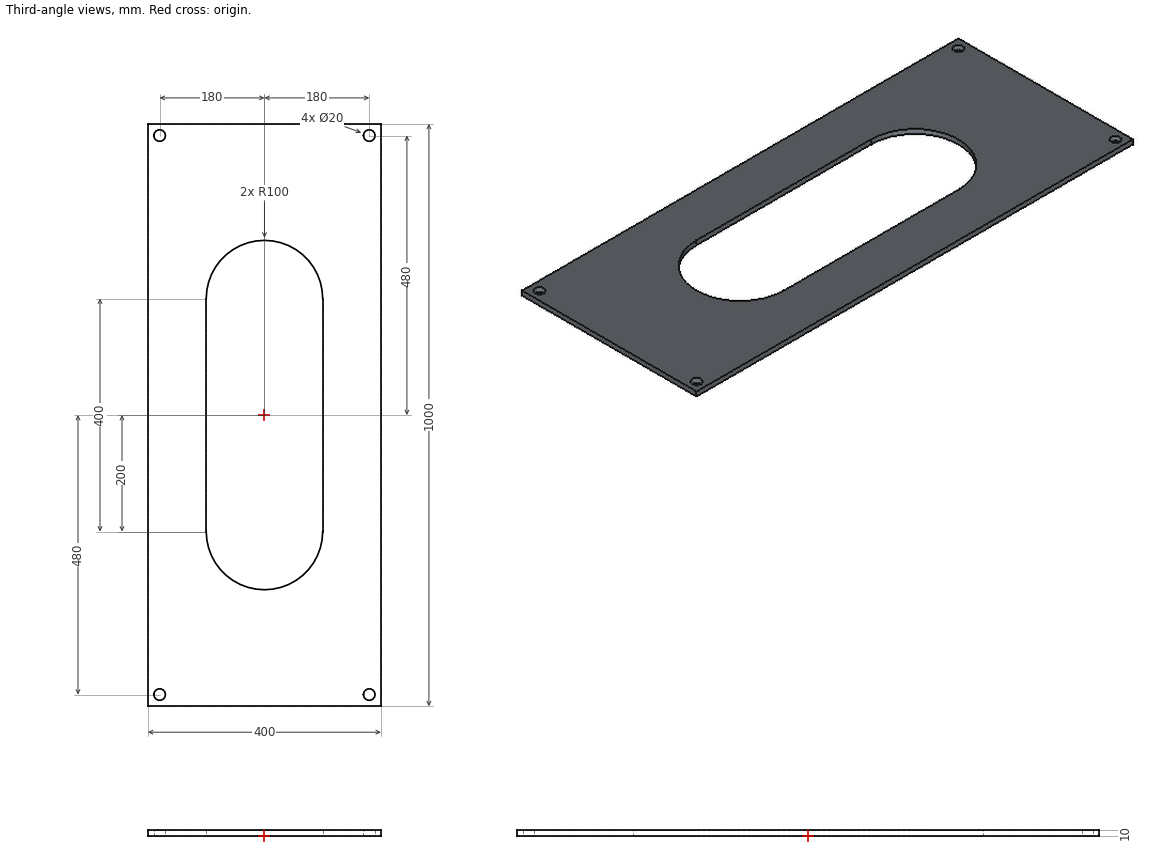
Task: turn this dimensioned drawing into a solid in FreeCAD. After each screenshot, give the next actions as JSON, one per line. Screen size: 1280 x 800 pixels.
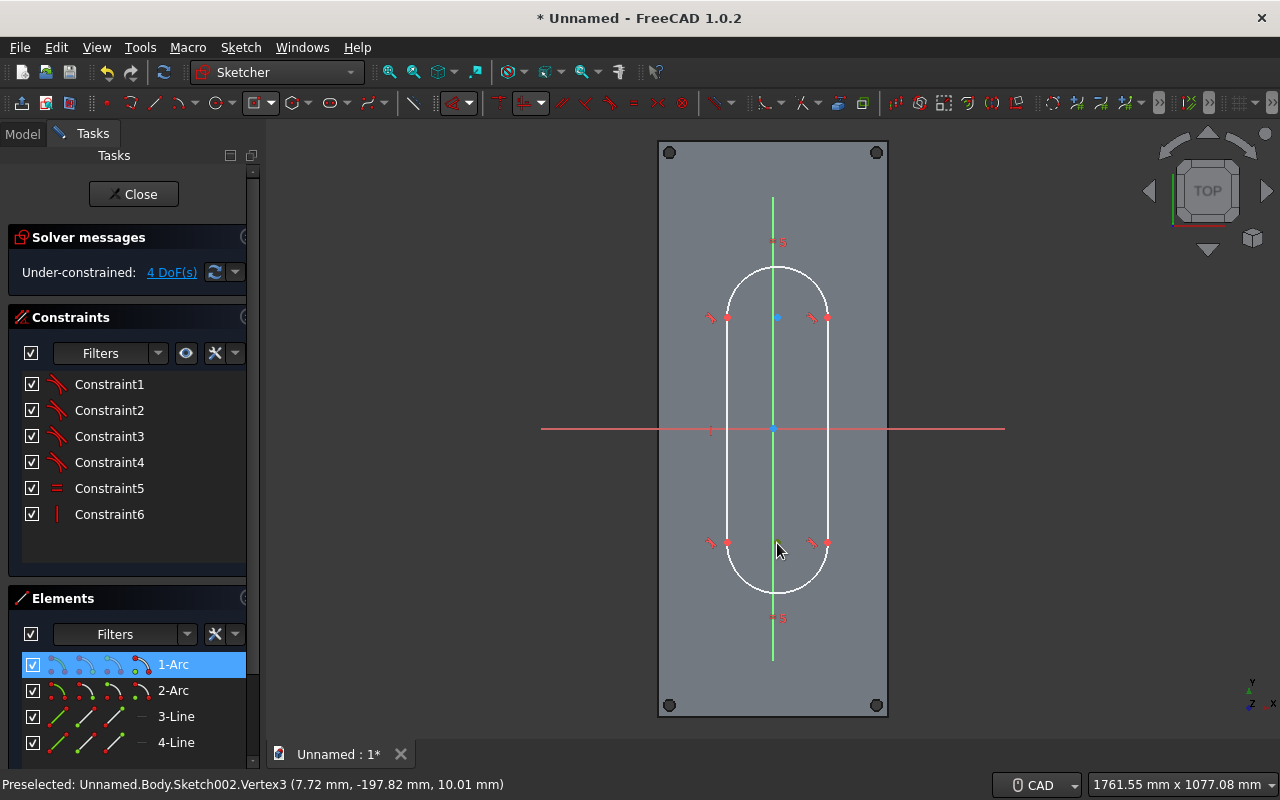
{"action": "left_click", "coordinate": [773, 630]}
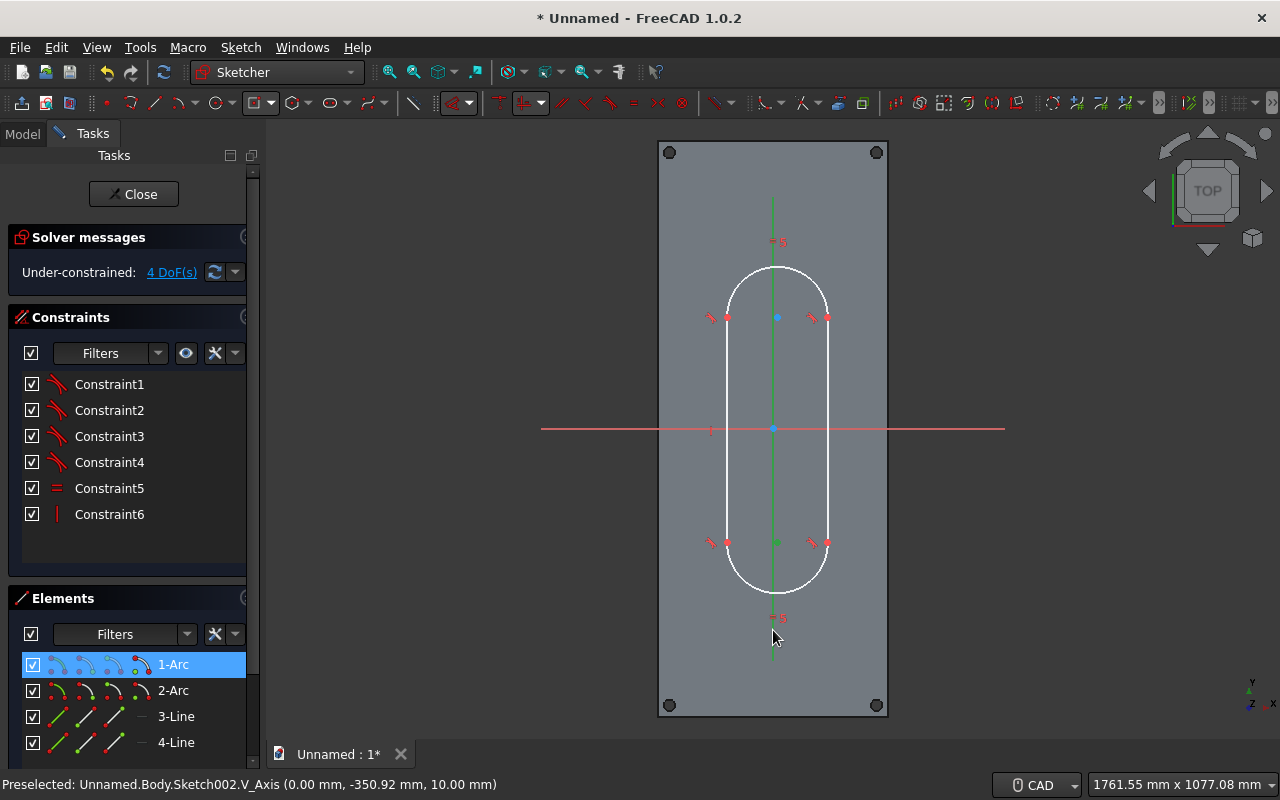
{"action": "left_click", "coordinate": [500, 104]}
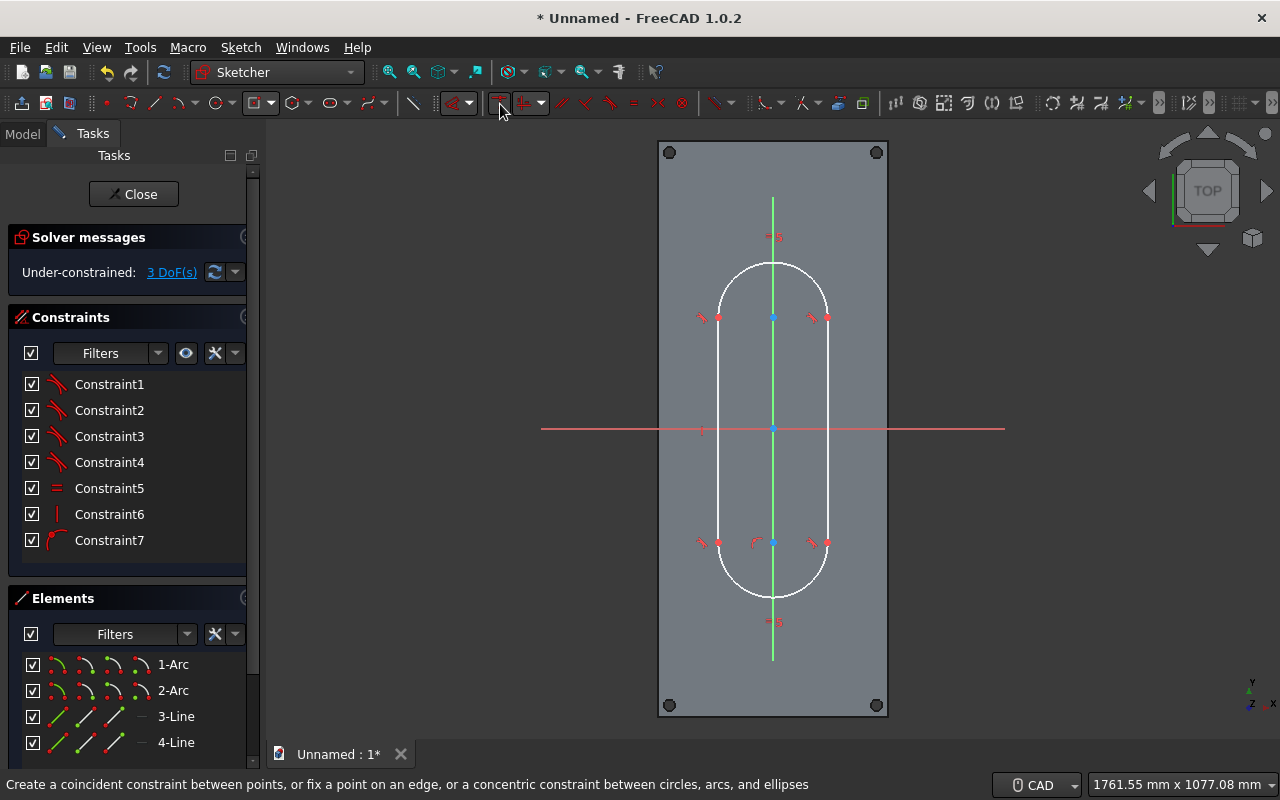
{"action": "left_click", "coordinate": [741, 587]}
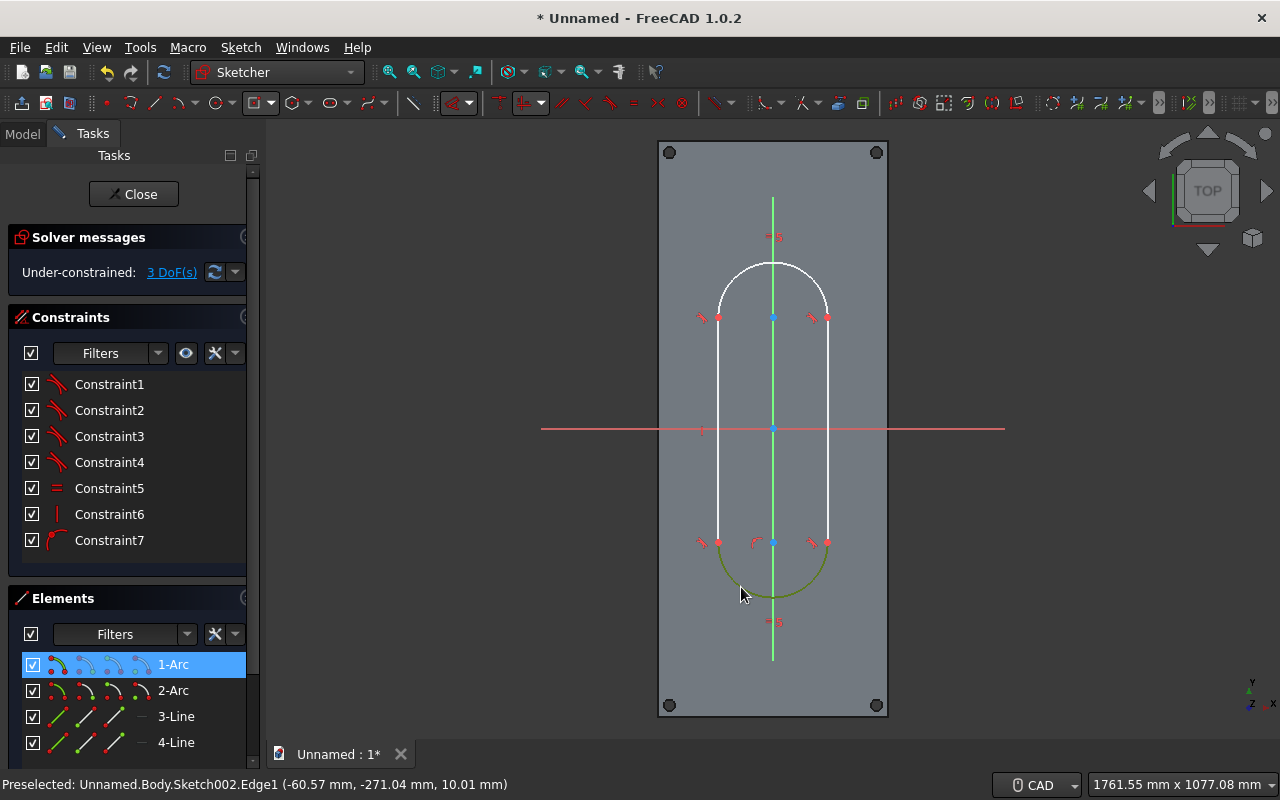
{"action": "left_click", "coordinate": [472, 104]}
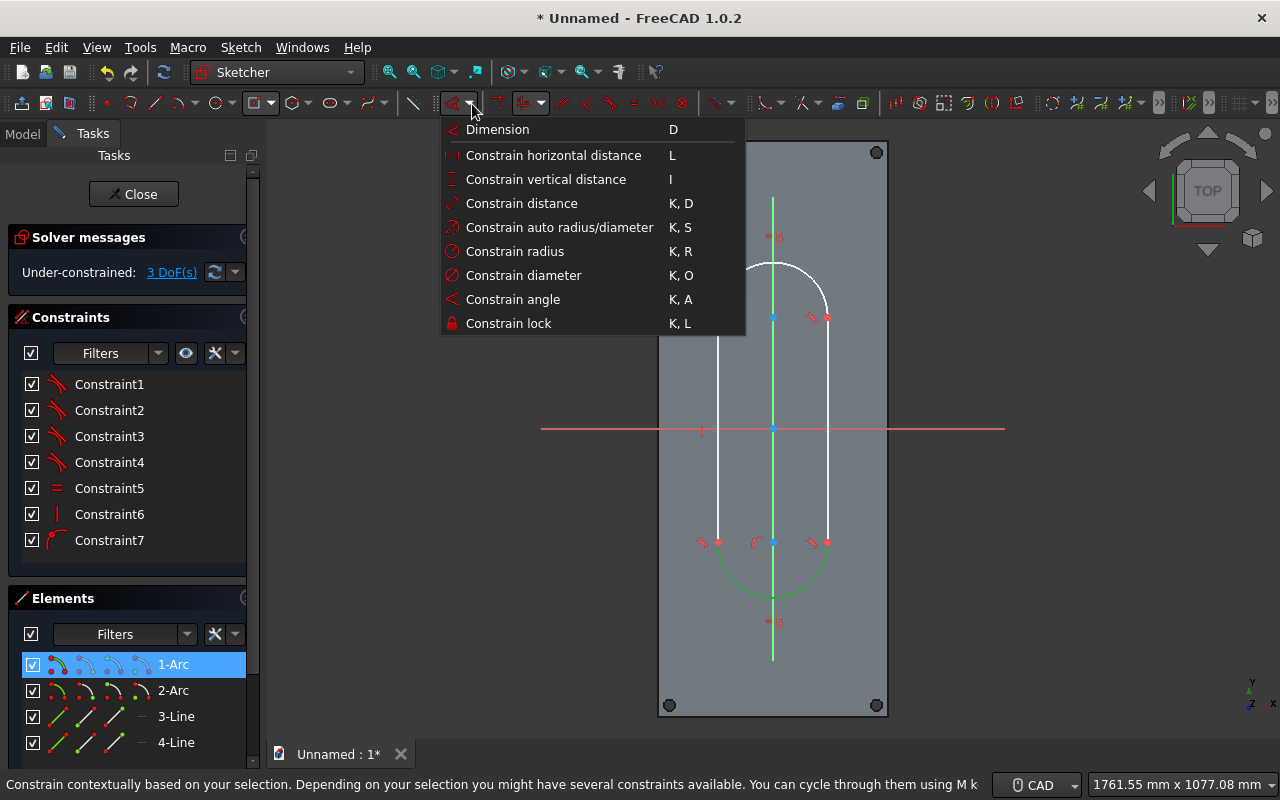
{"action": "left_click", "coordinate": [593, 251]}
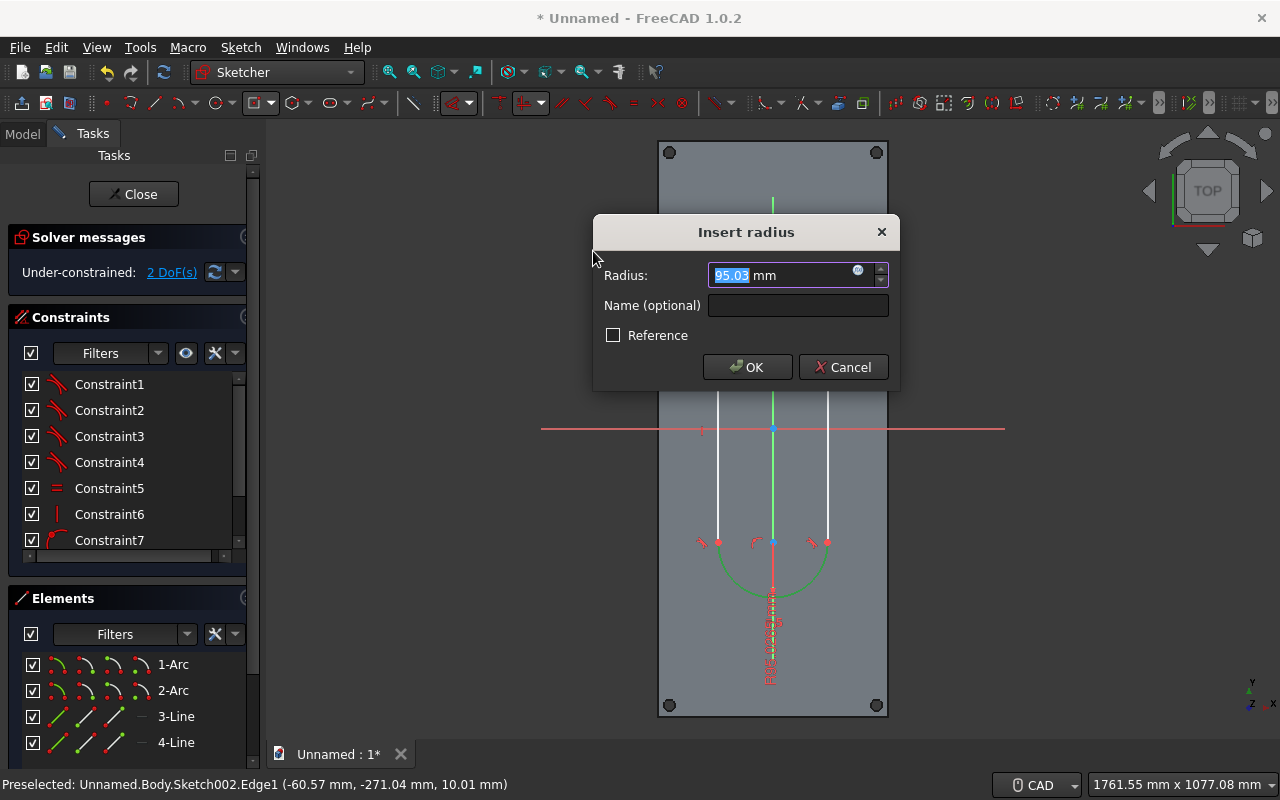
{"action": "type", "text": "100"}
{"action": "key", "text": "Return"}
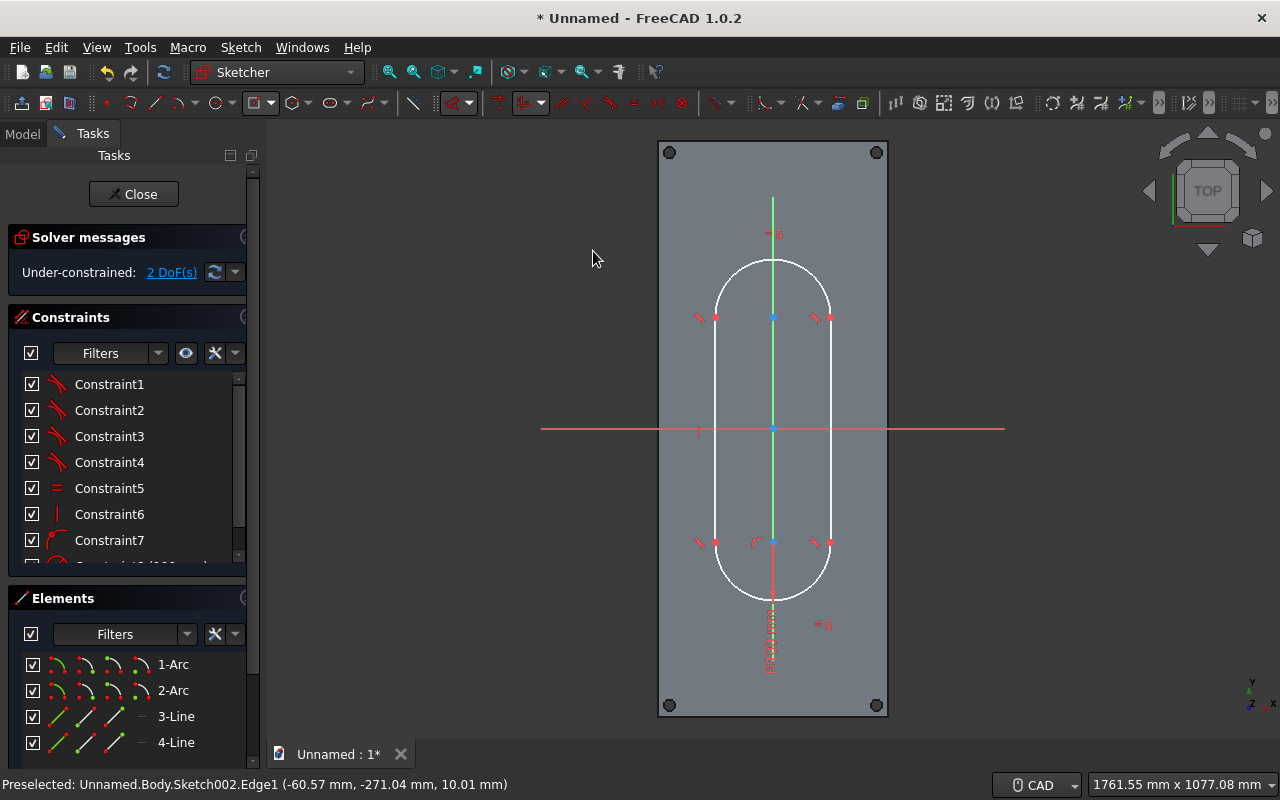
{"action": "left_click", "coordinate": [715, 475]}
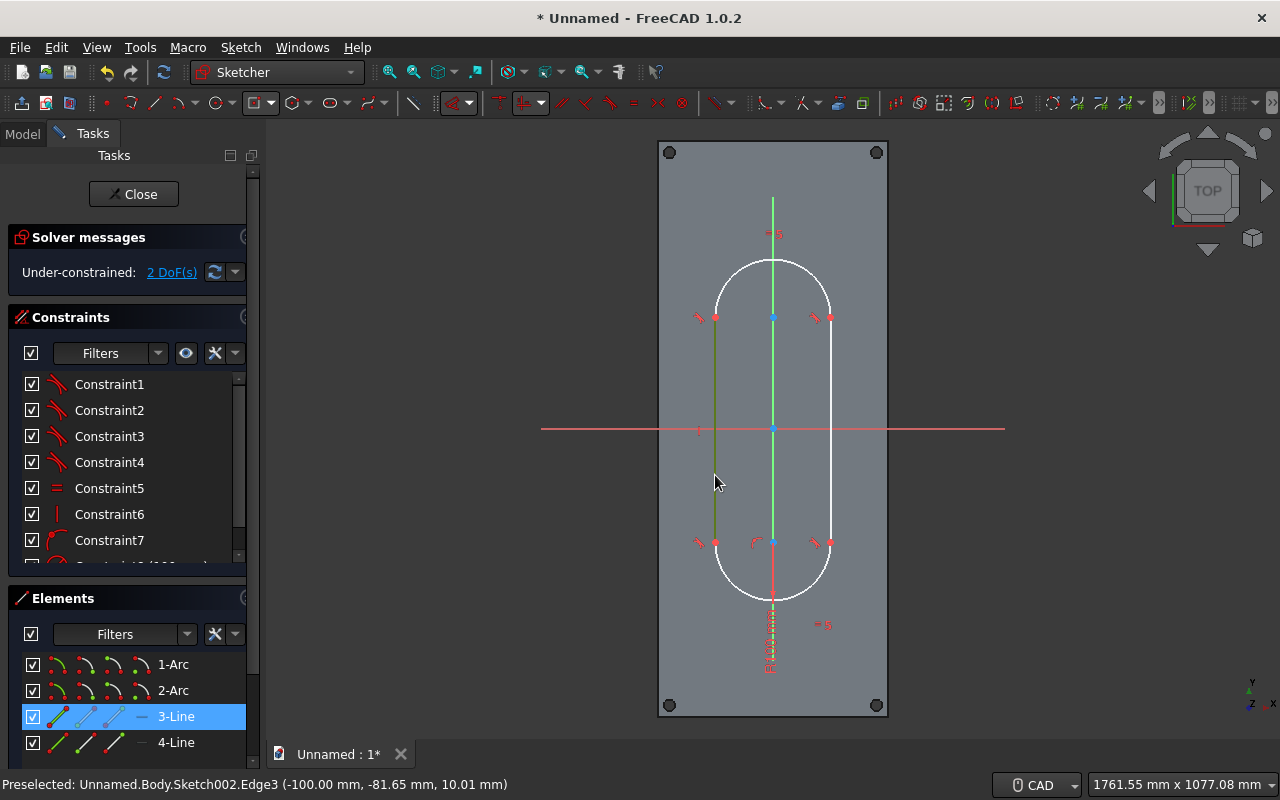
{"action": "left_click", "coordinate": [472, 104]}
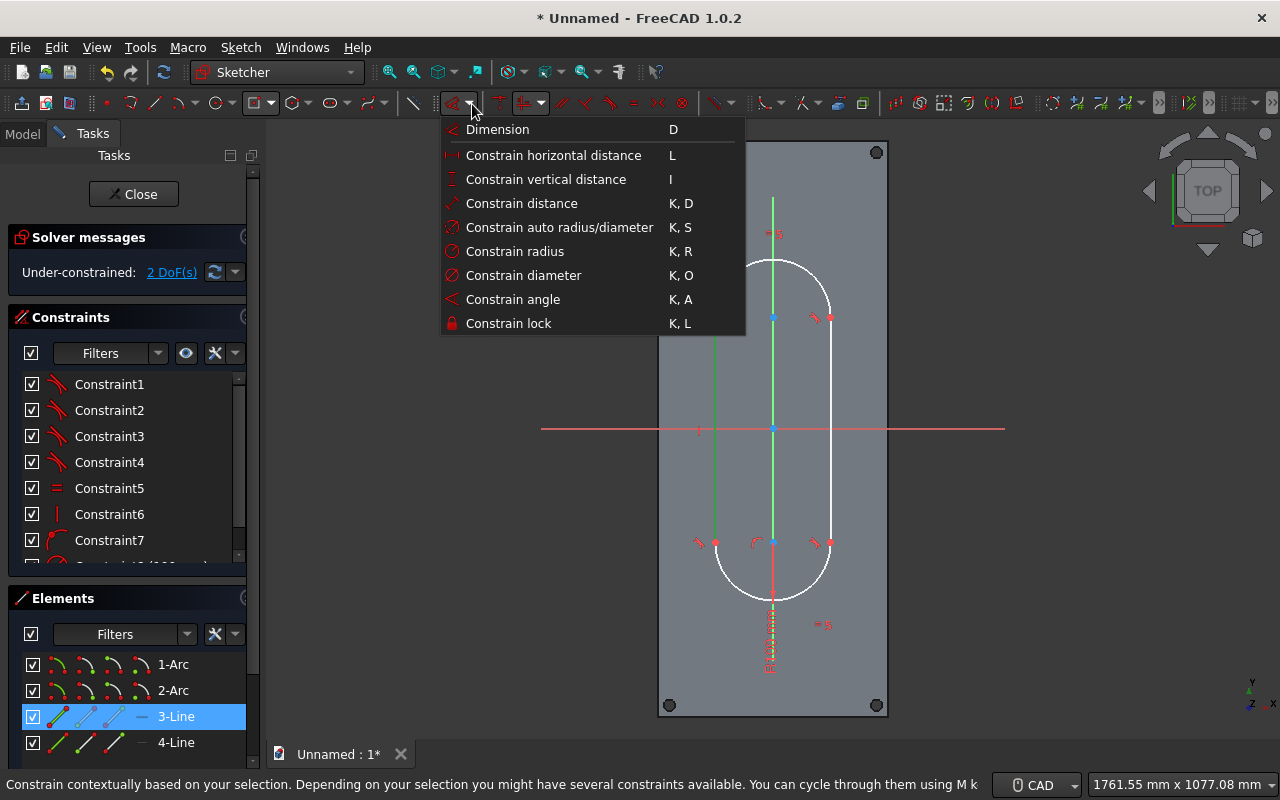
{"action": "left_click", "coordinate": [593, 179]}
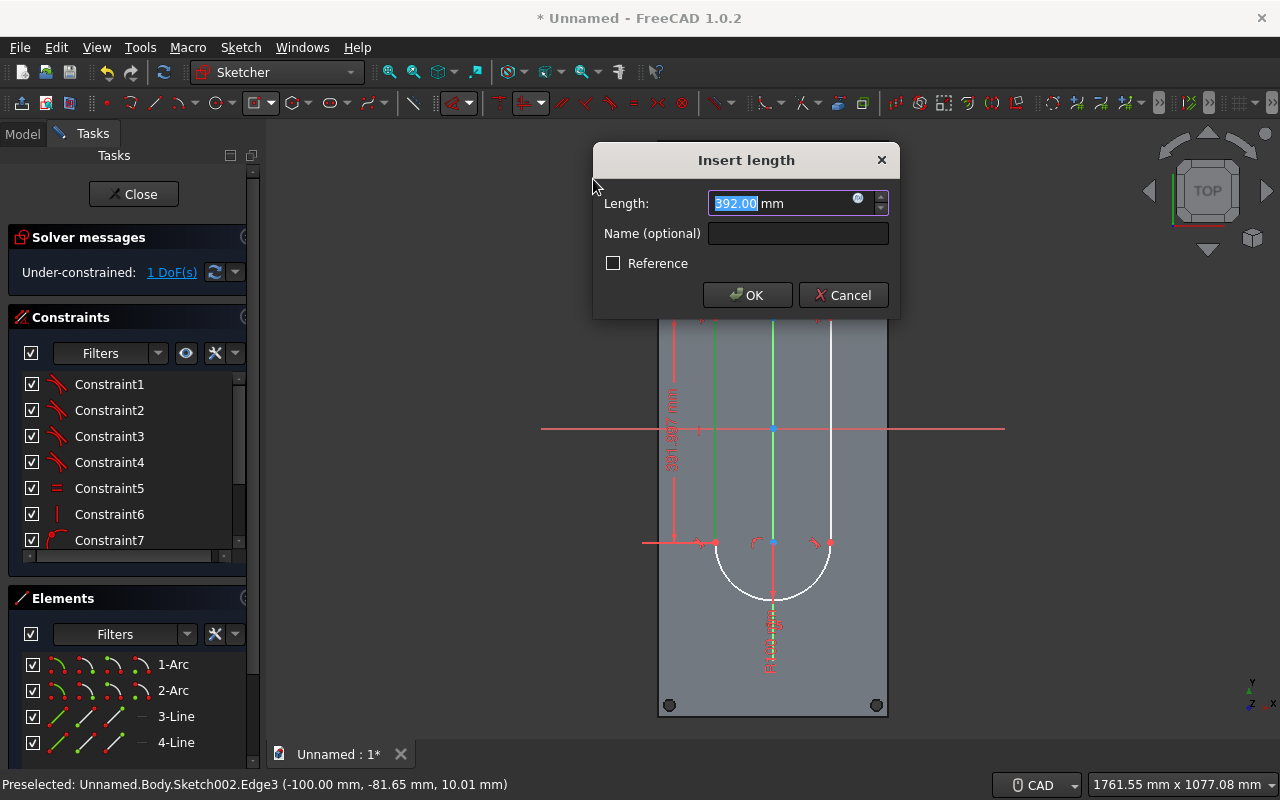
{"action": "type", "text": "400"}
{"action": "key", "text": "Return"}